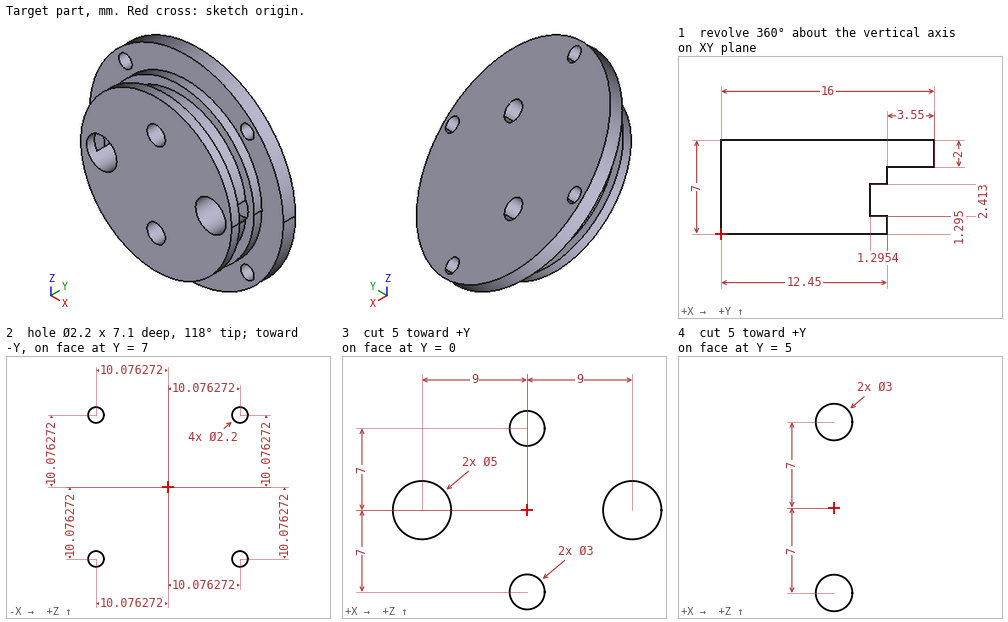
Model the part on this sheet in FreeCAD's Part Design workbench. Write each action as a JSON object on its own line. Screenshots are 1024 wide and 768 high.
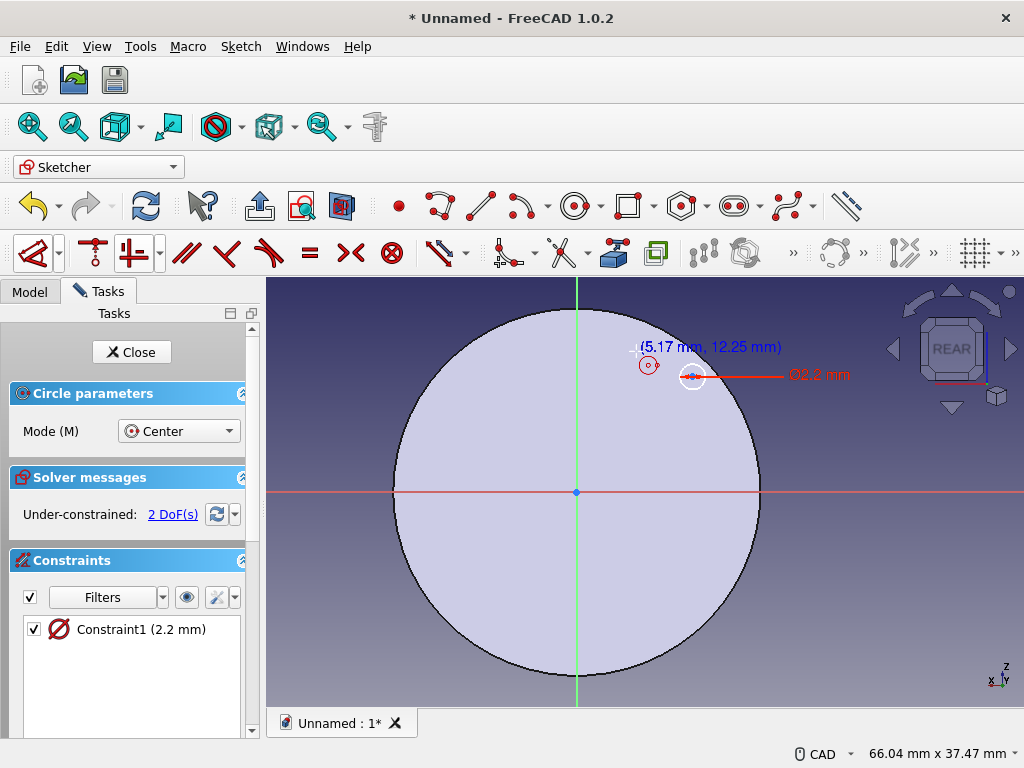
{"action": "scroll", "coordinate": [692, 608], "scroll_direction": "up", "scroll_amount": 3}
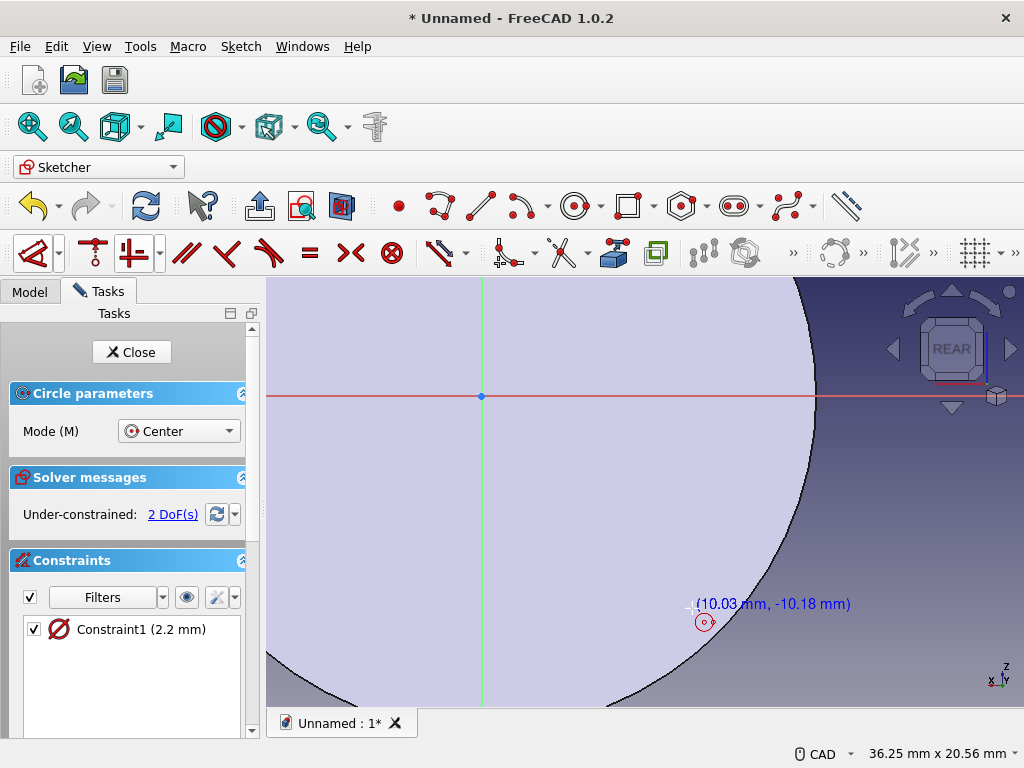
{"action": "left_click", "coordinate": [692, 607]}
{"action": "mouse_move", "coordinate": [709, 591]}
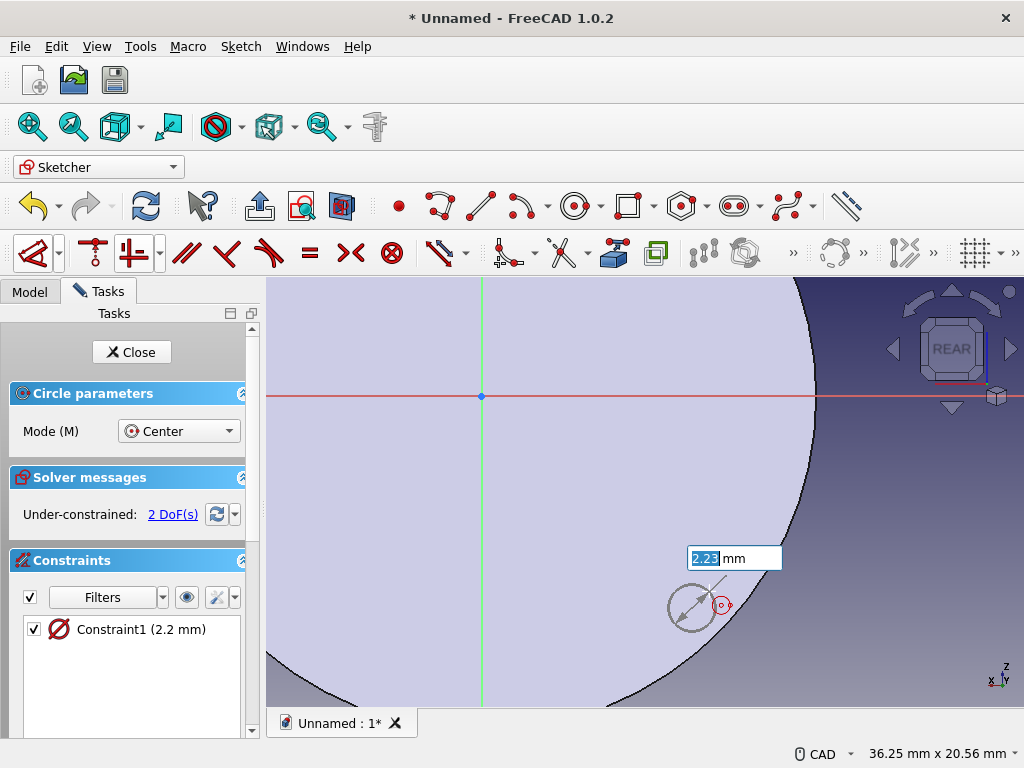
{"action": "type", "text": "2.2"}
{"action": "key", "text": "Return"}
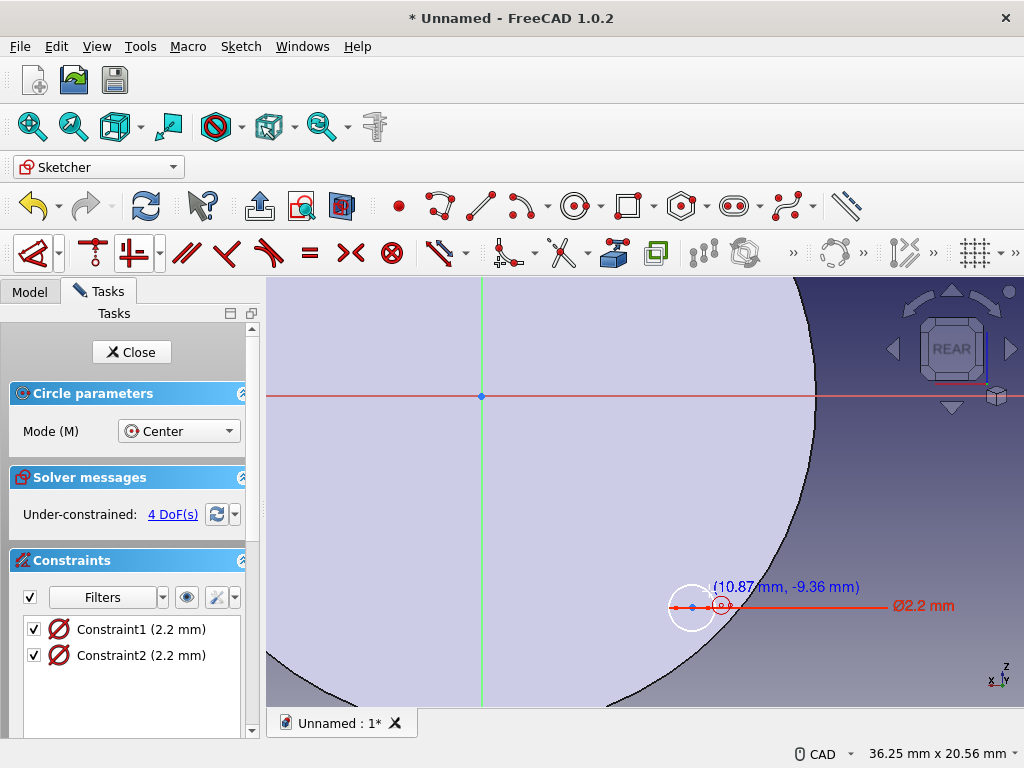
{"action": "scroll", "coordinate": [692, 608], "scroll_direction": "down", "scroll_amount": 3}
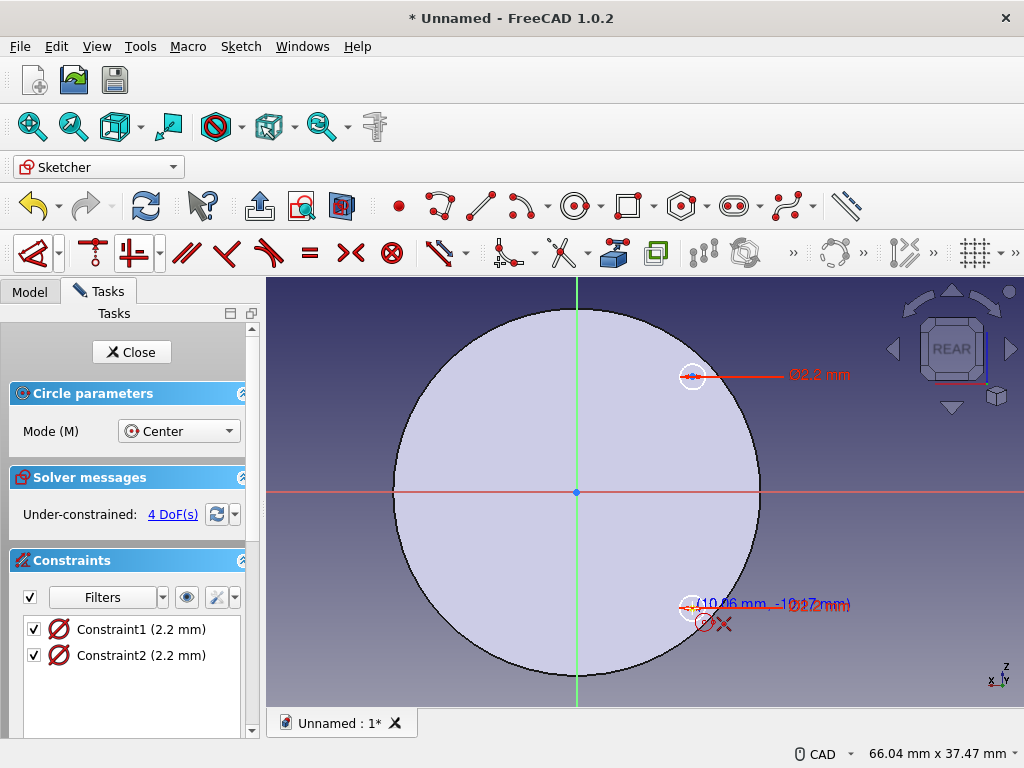
{"action": "scroll", "coordinate": [461, 608], "scroll_direction": "up", "scroll_amount": 3}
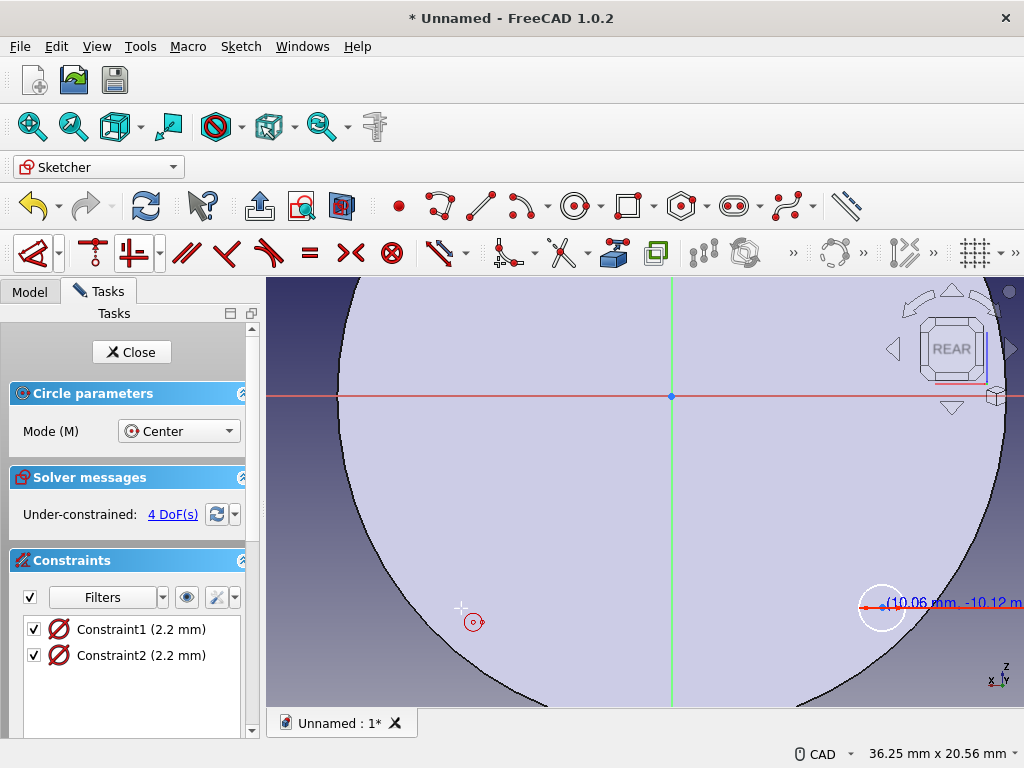
{"action": "left_click", "coordinate": [461, 607]}
{"action": "mouse_move", "coordinate": [477, 591]}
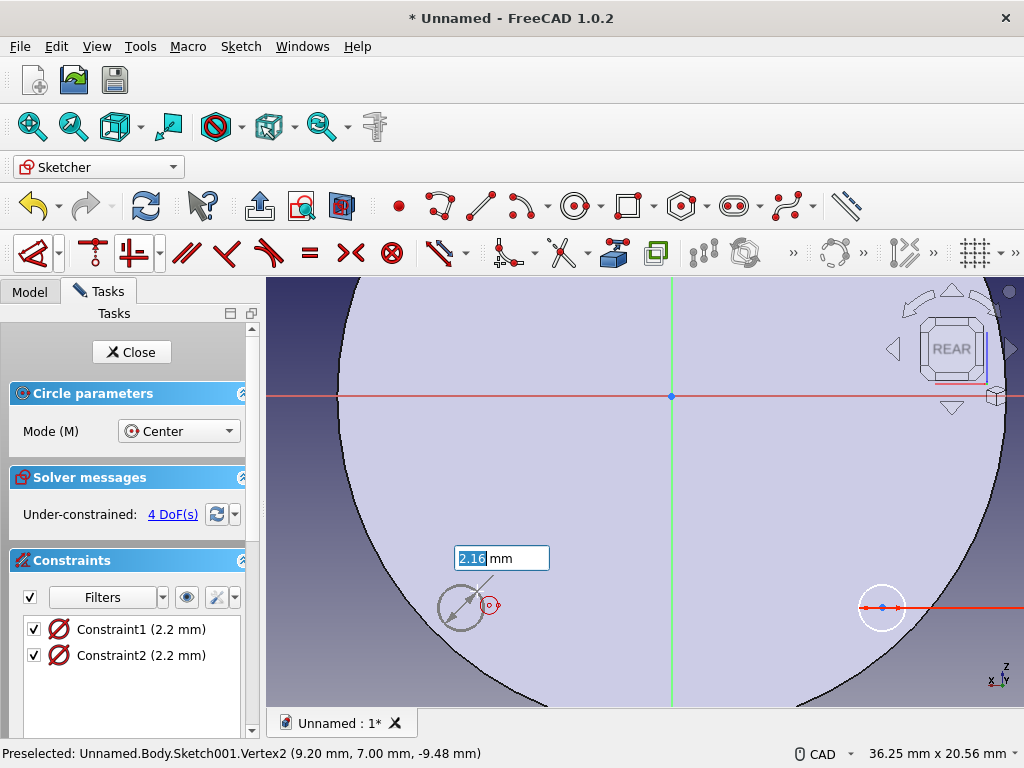
{"action": "type", "text": "2.2"}
{"action": "key", "text": "Return"}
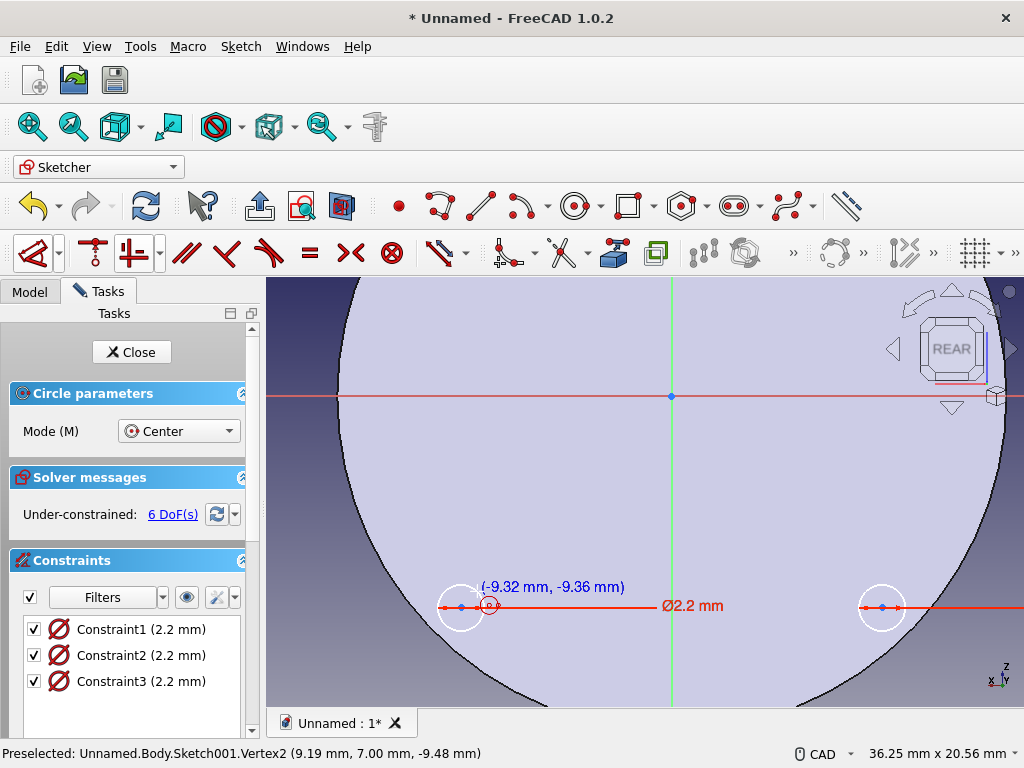
{"action": "scroll", "coordinate": [460, 608], "scroll_direction": "down", "scroll_amount": 3}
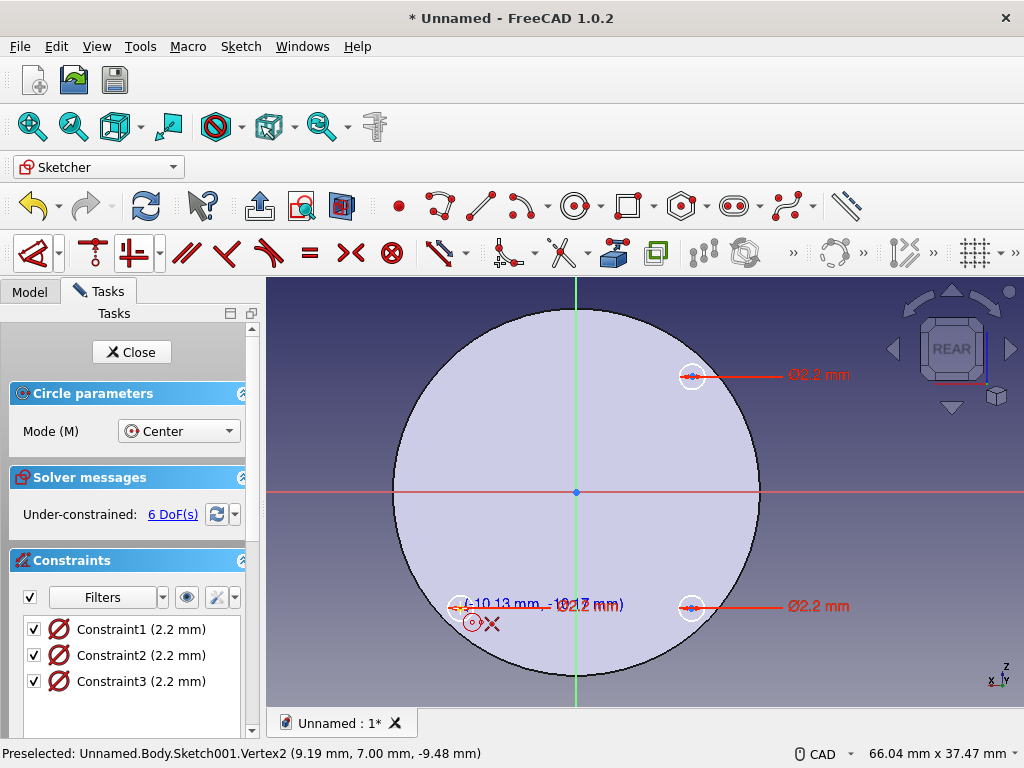
{"action": "scroll", "coordinate": [461, 377], "scroll_direction": "up", "scroll_amount": 3}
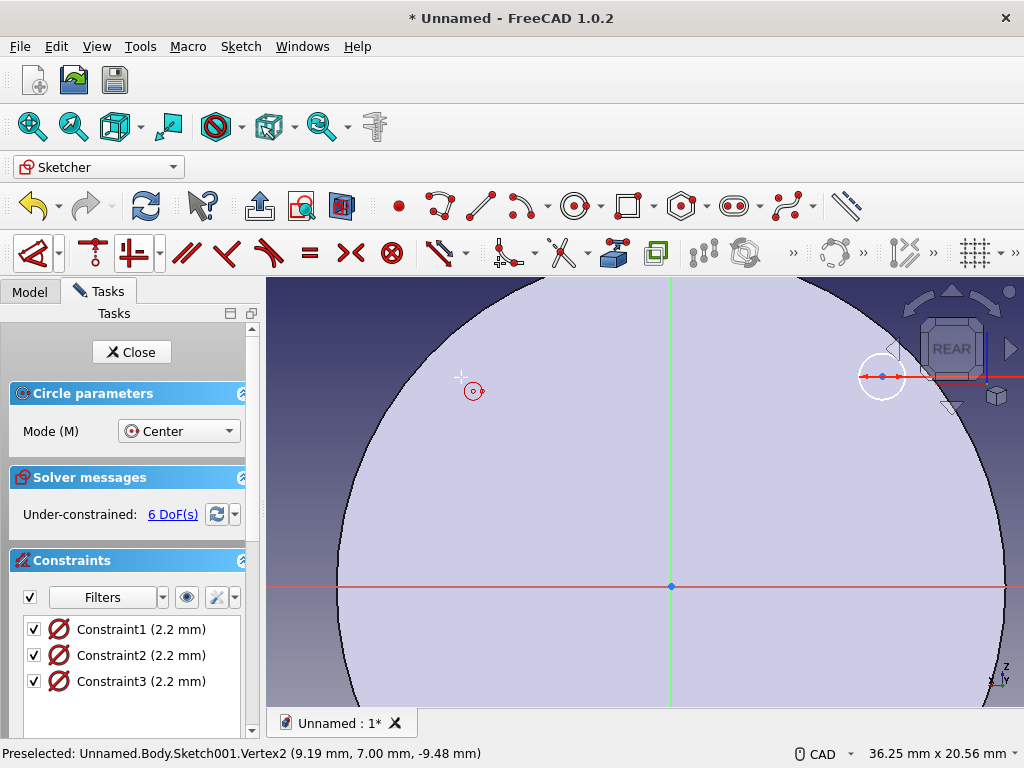
{"action": "left_click", "coordinate": [460, 376]}
{"action": "mouse_move", "coordinate": [477, 360]}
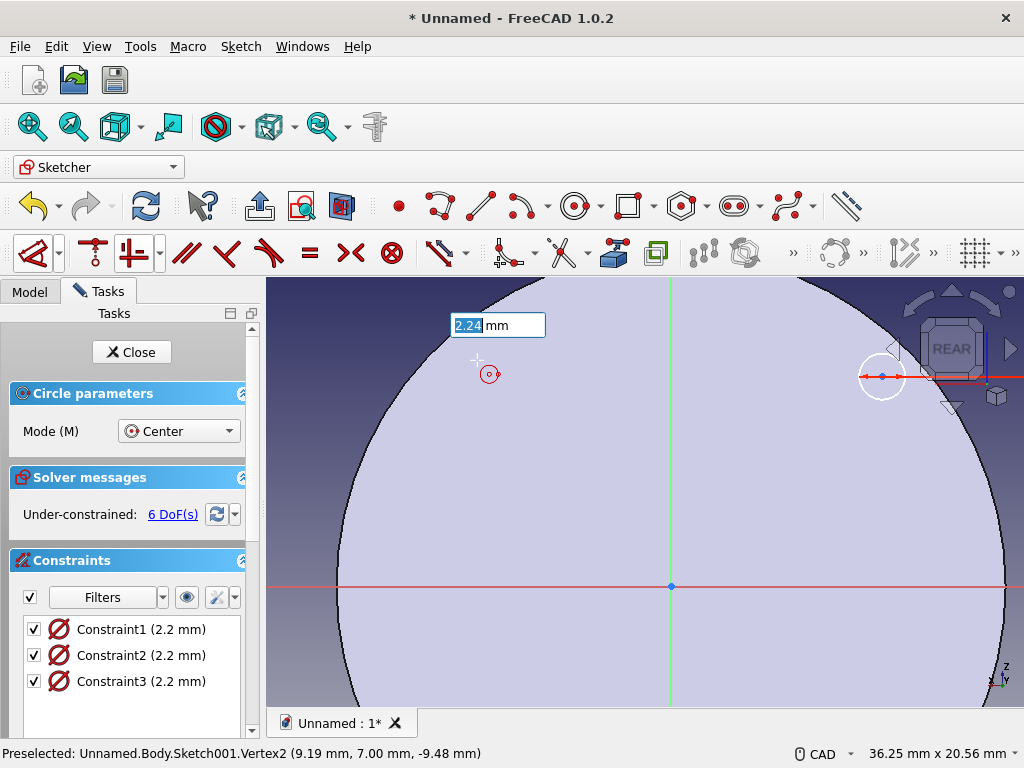
{"action": "type", "text": "2.2"}
{"action": "key", "text": "Return"}
{"action": "key", "text": "Escape"}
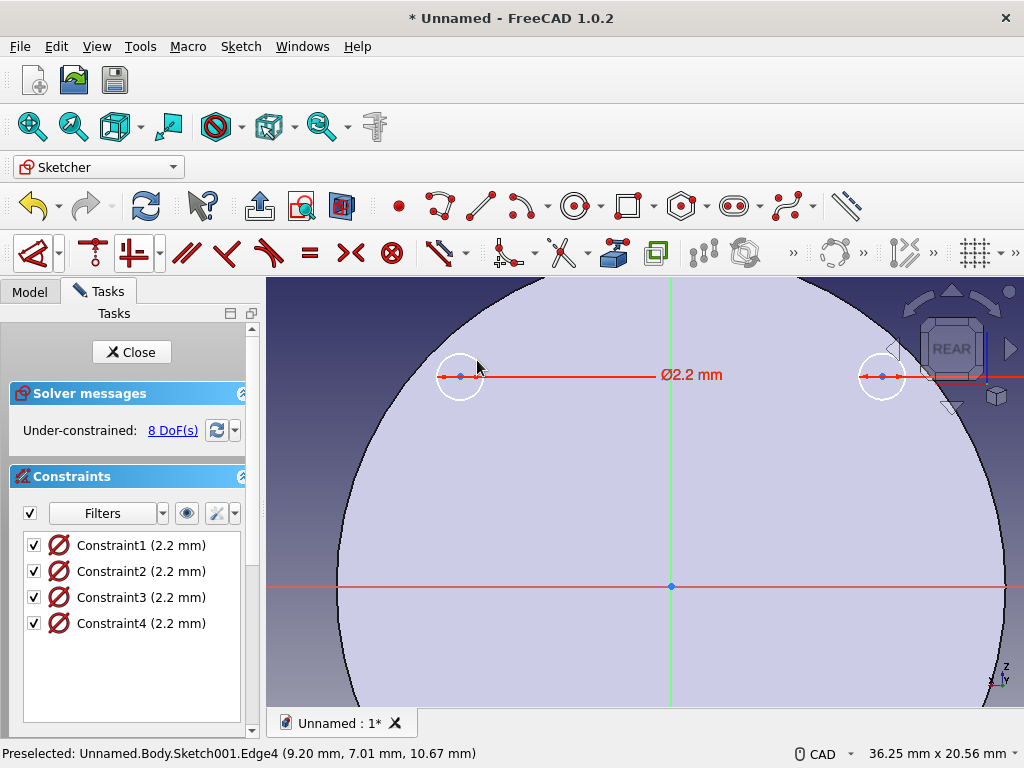
{"action": "scroll", "coordinate": [461, 377], "scroll_direction": "down", "scroll_amount": 3}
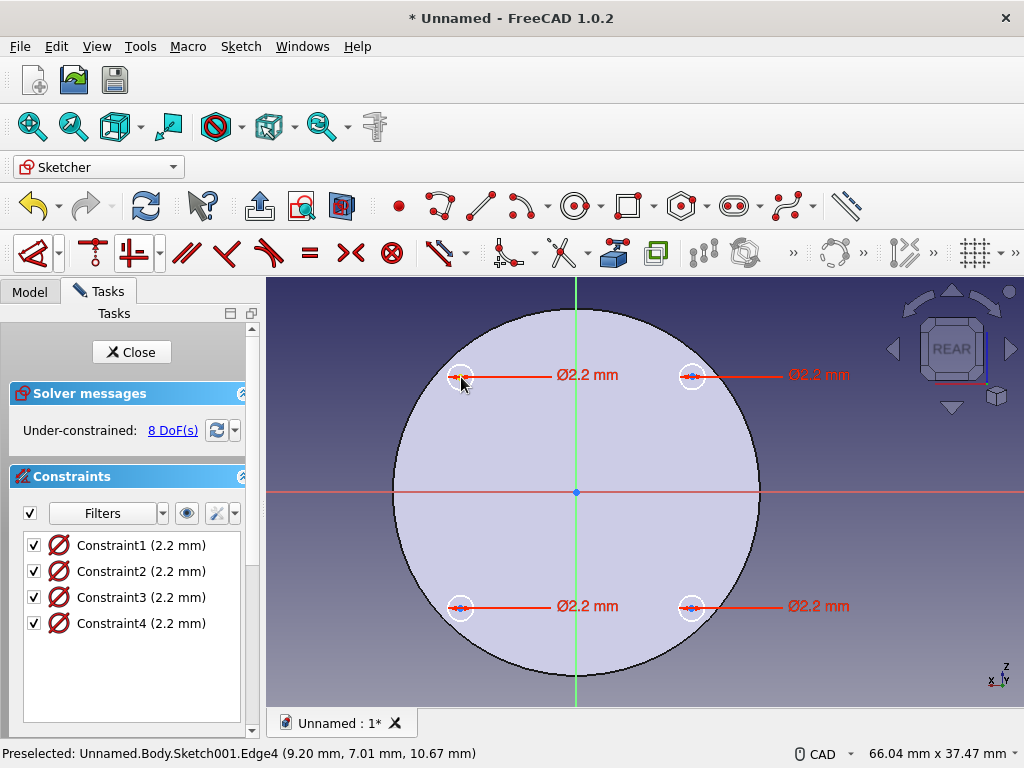
{"action": "left_click", "coordinate": [692, 377]}